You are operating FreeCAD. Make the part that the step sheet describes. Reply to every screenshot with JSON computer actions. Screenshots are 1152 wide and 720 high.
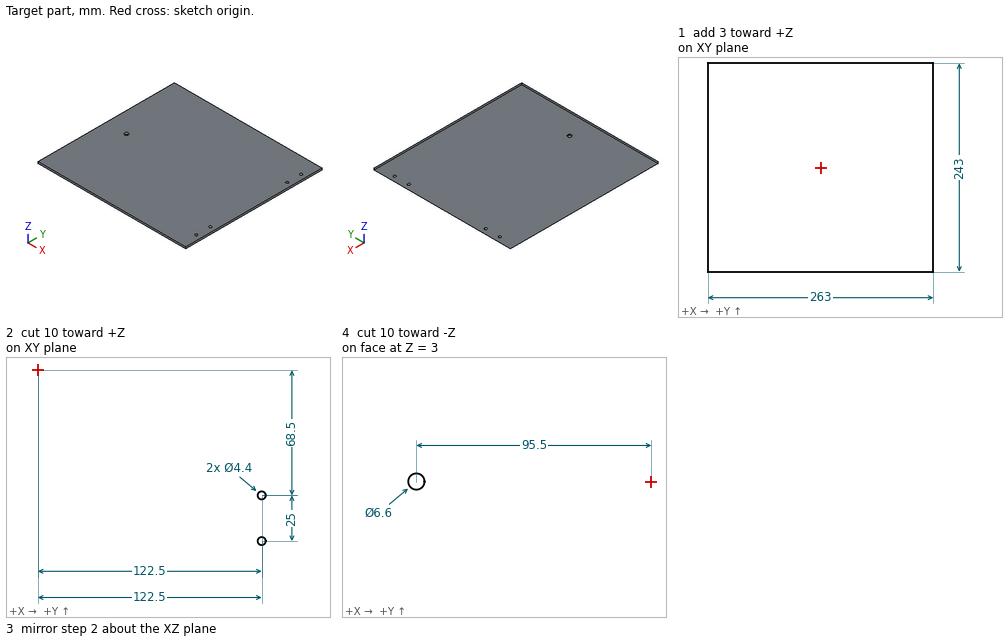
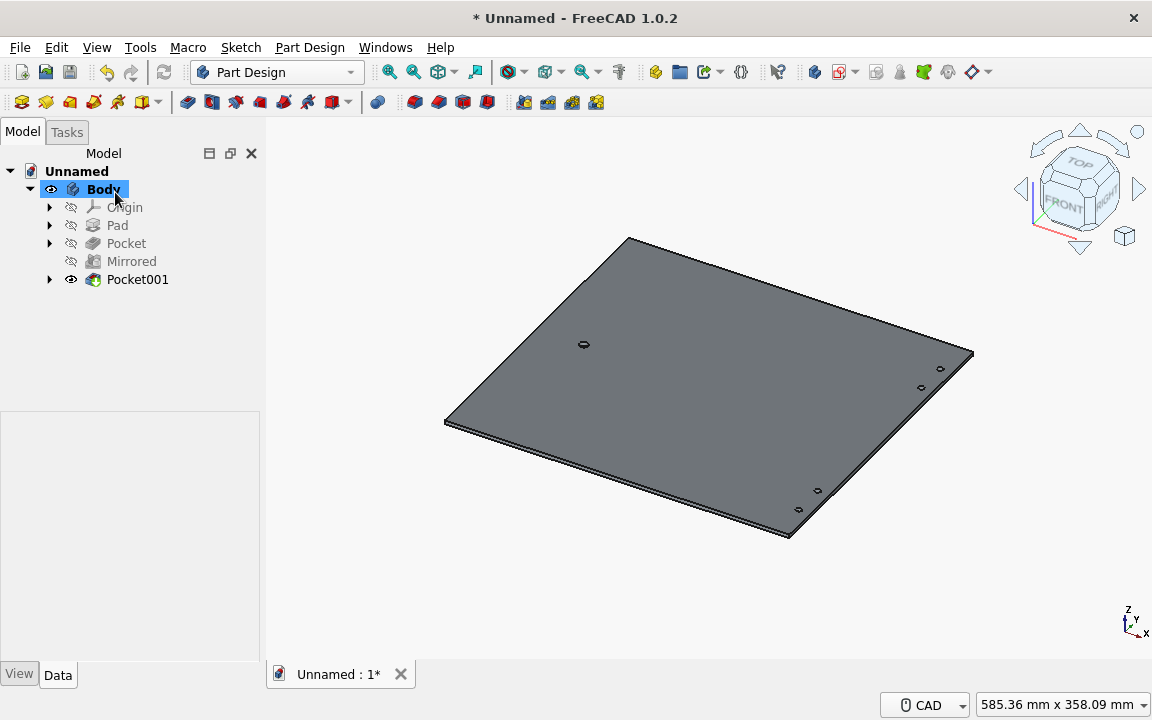
{"action": "key", "text": "0"}